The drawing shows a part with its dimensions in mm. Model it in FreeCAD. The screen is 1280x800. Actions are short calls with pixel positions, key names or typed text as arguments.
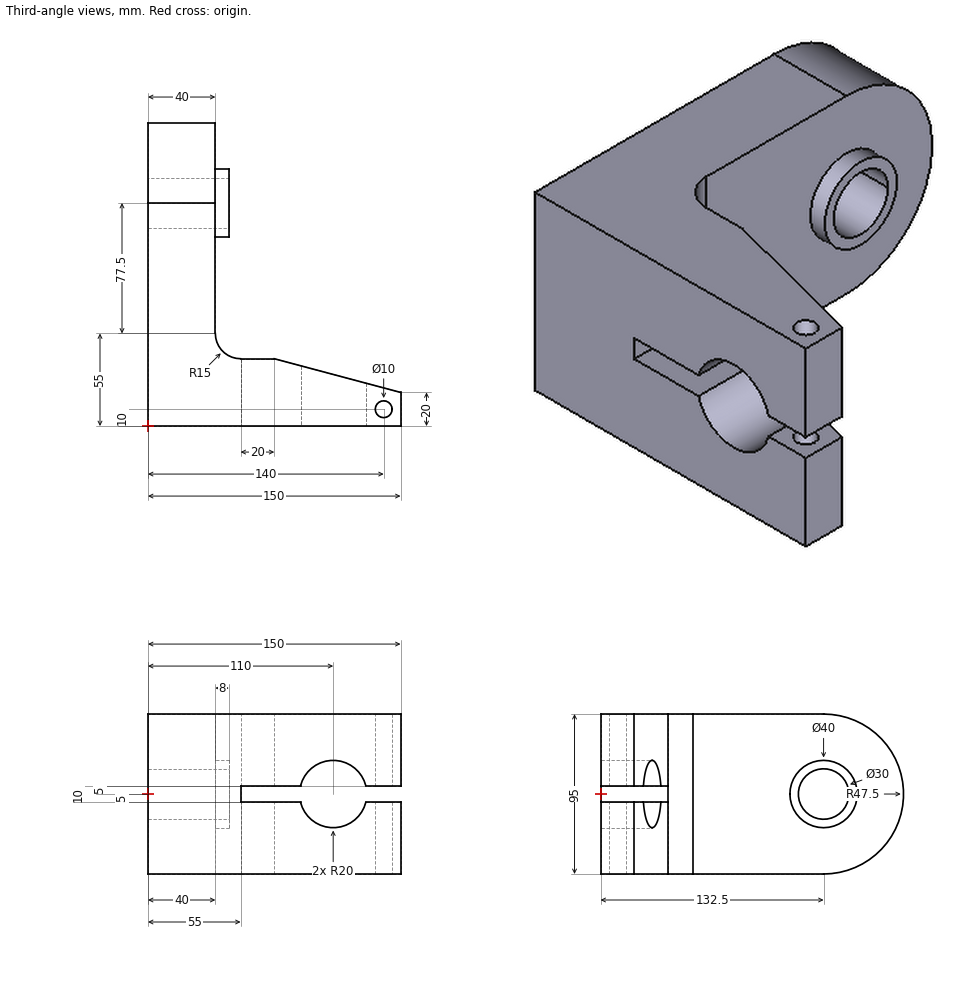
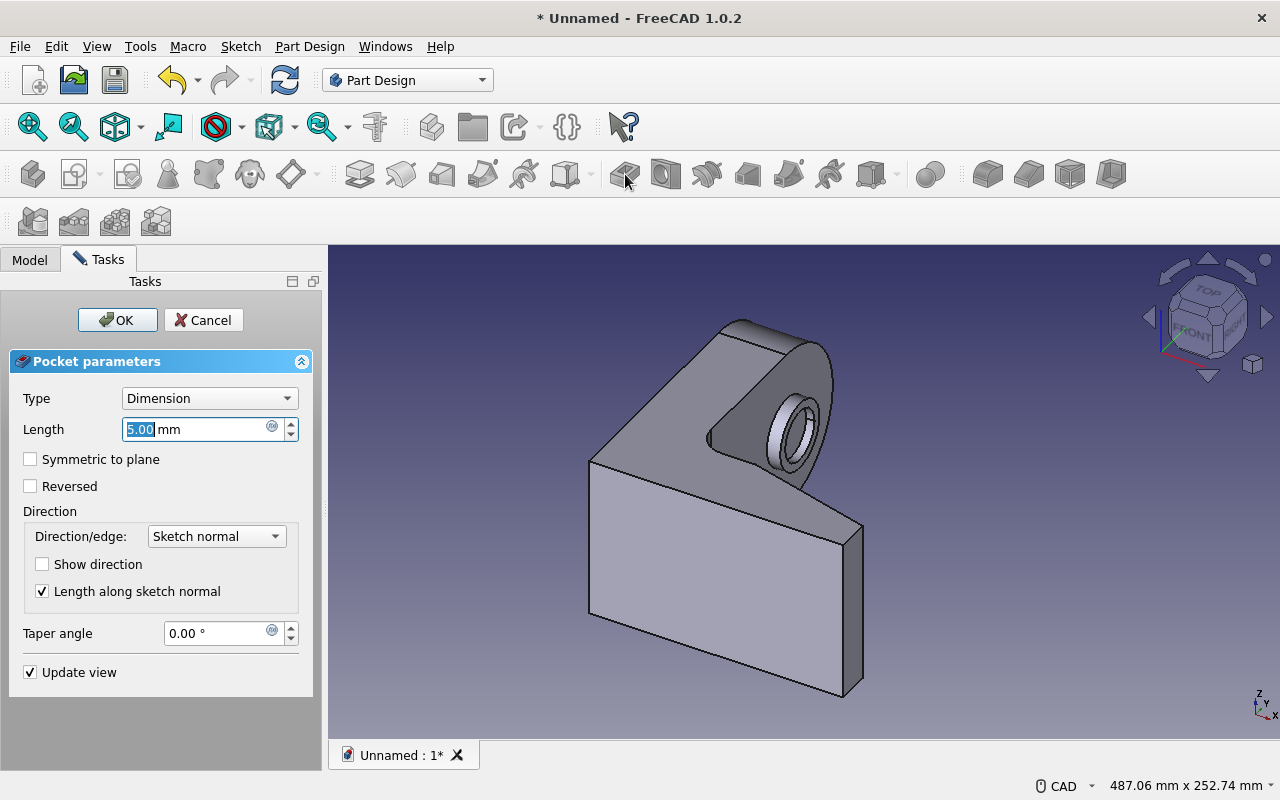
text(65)
key(Tab)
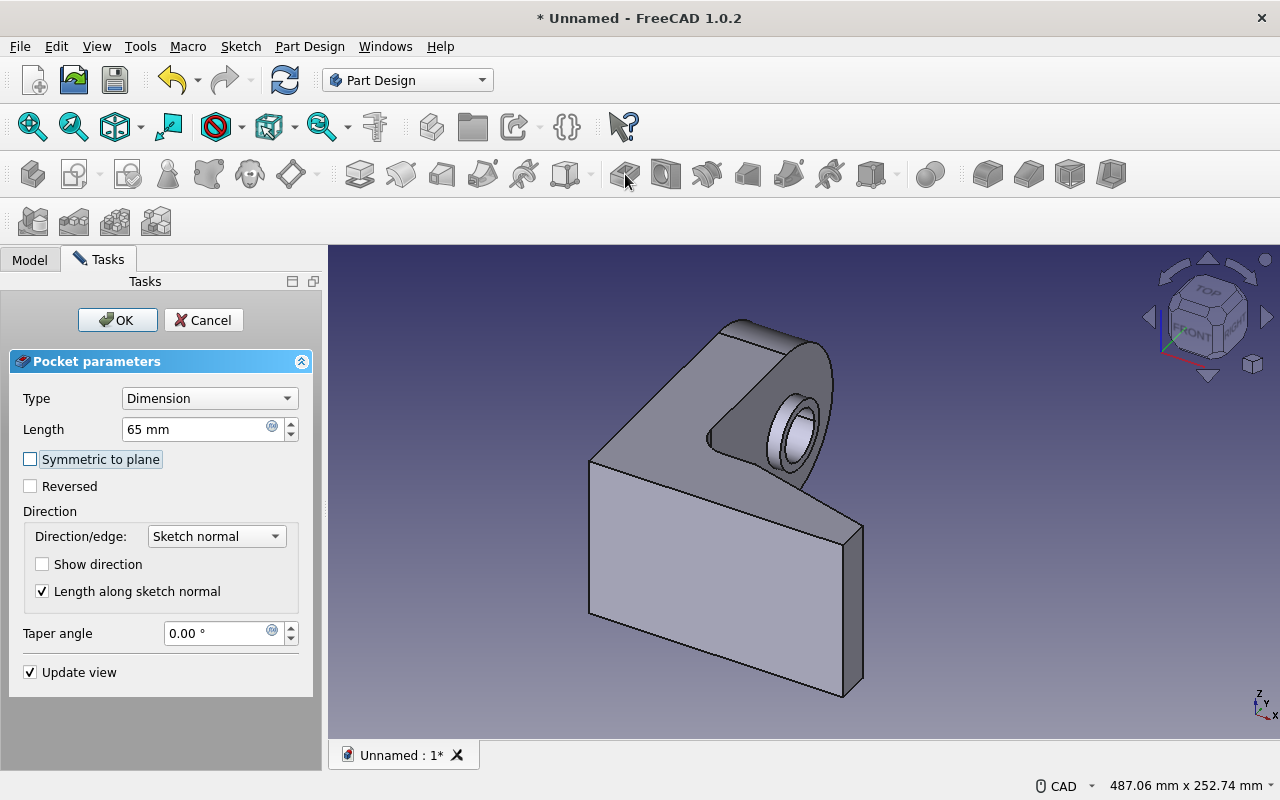
click(118, 320)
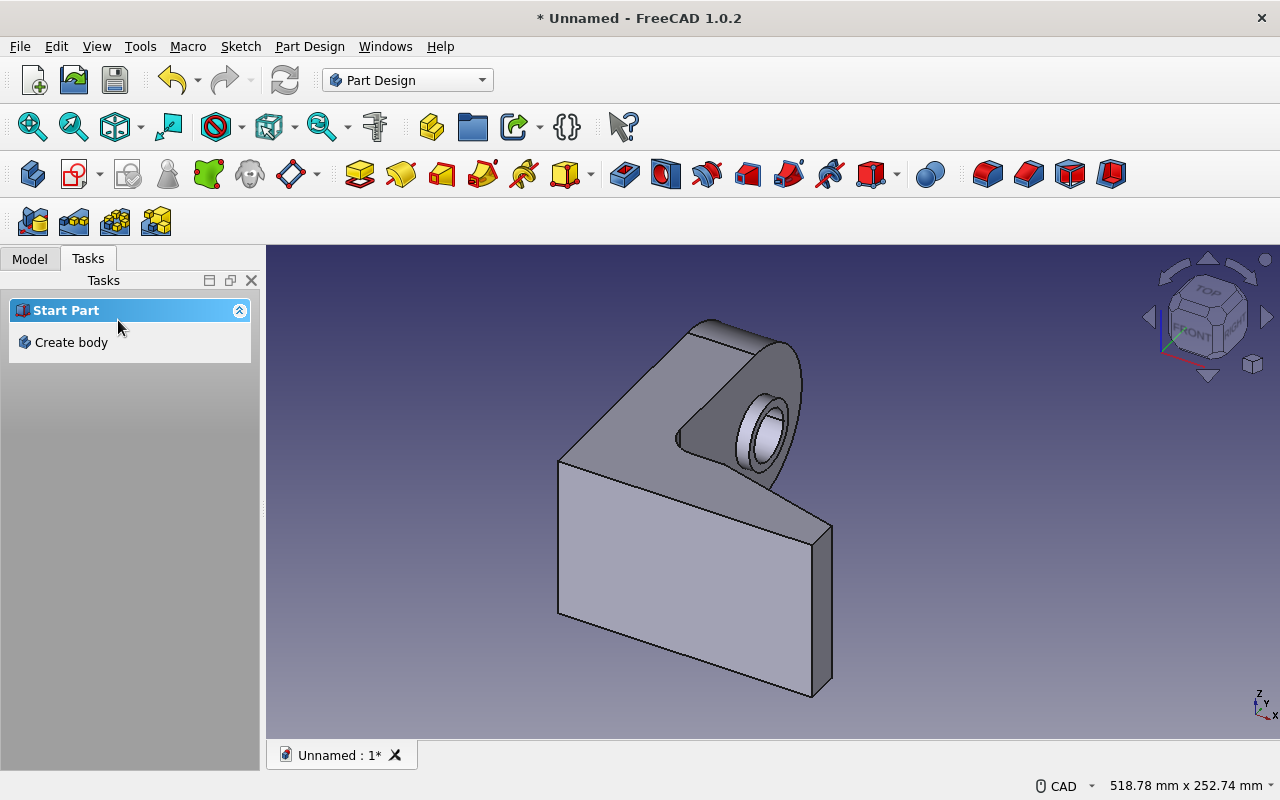
key(4)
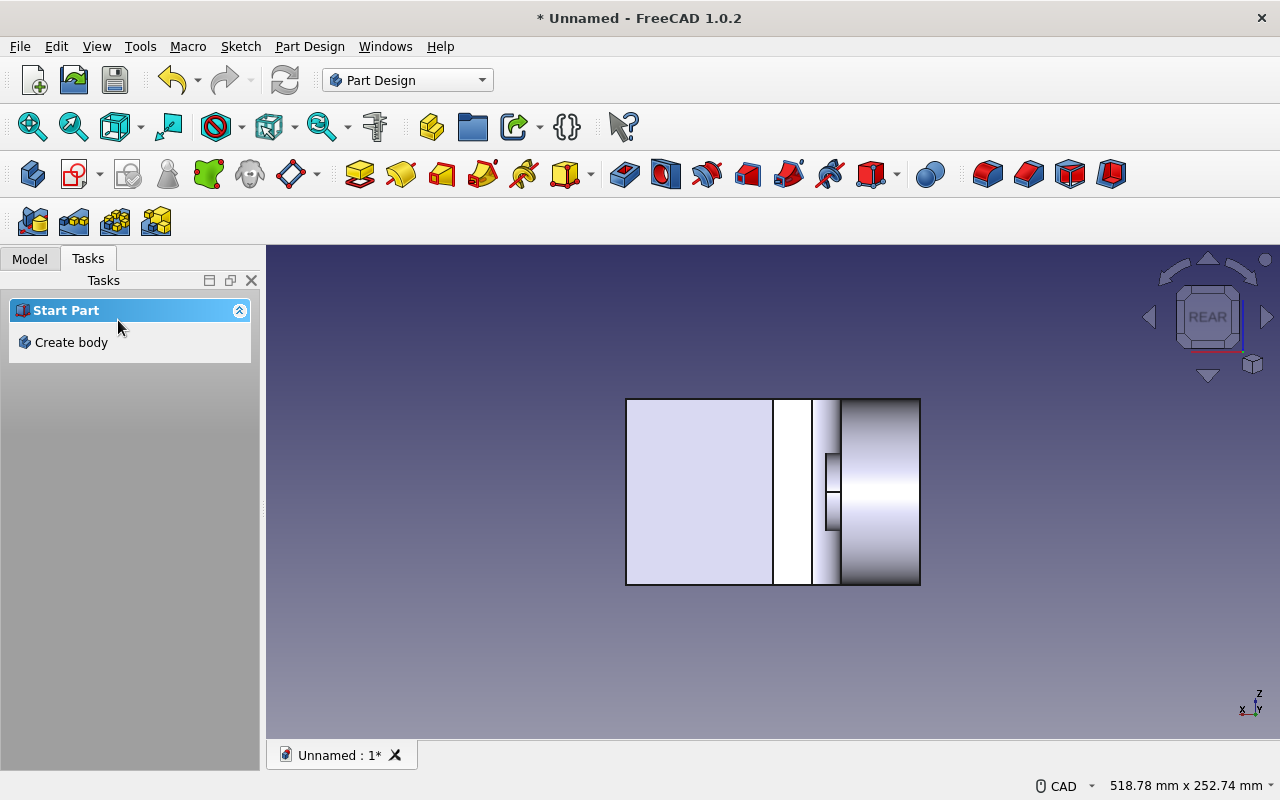
click(33, 128)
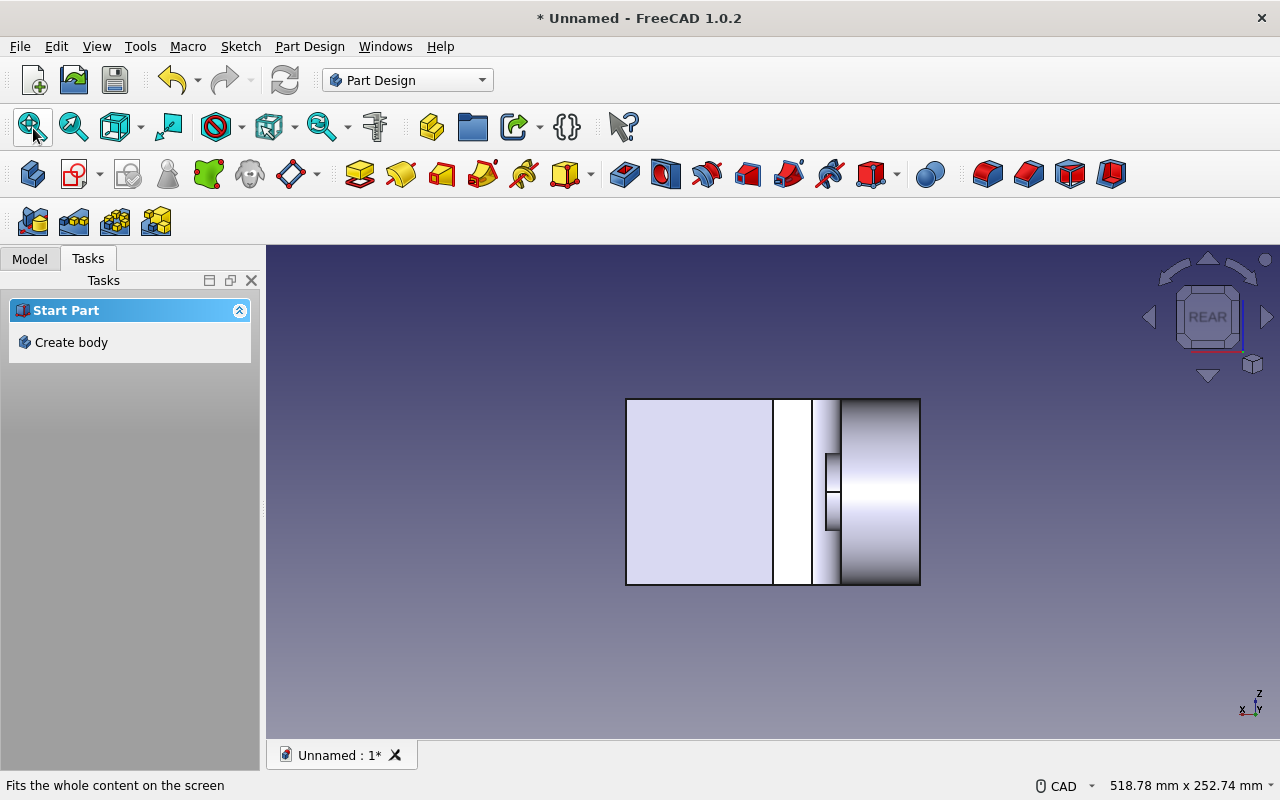
click(793, 438)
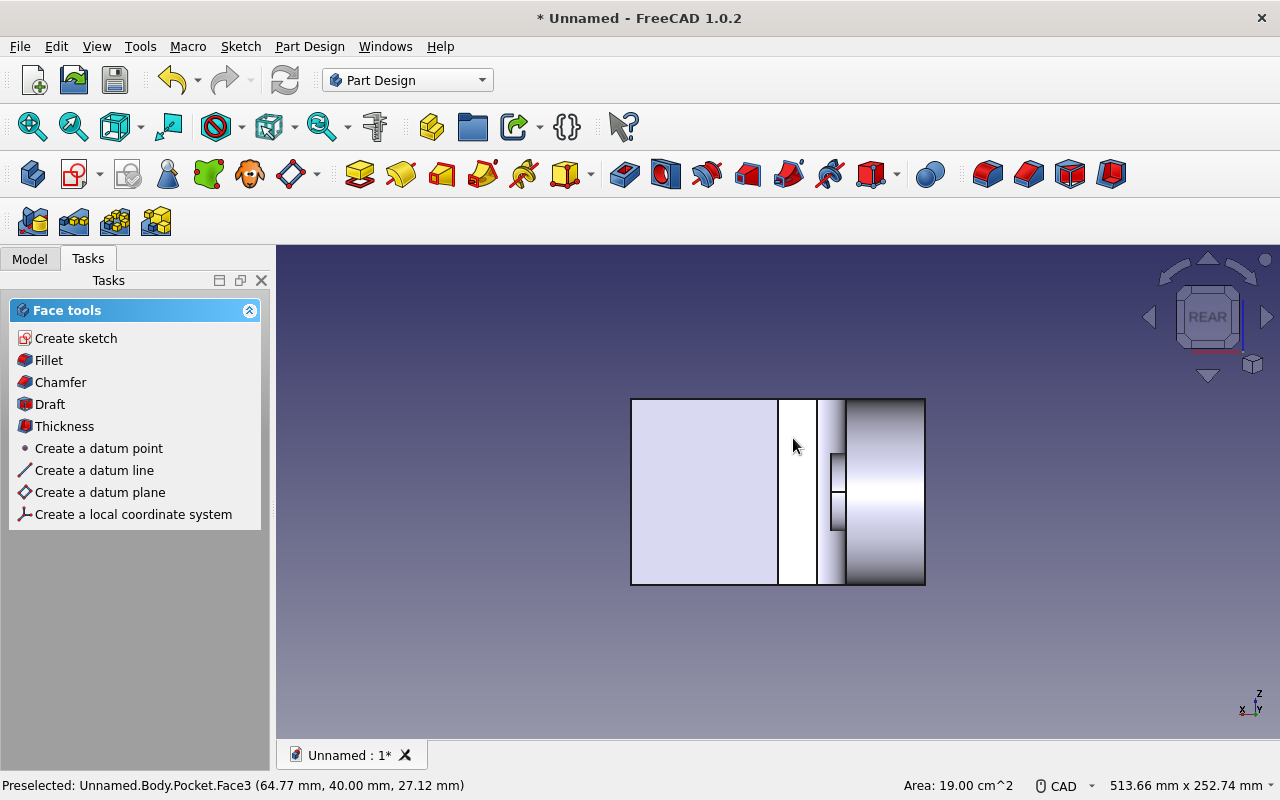
click(74, 174)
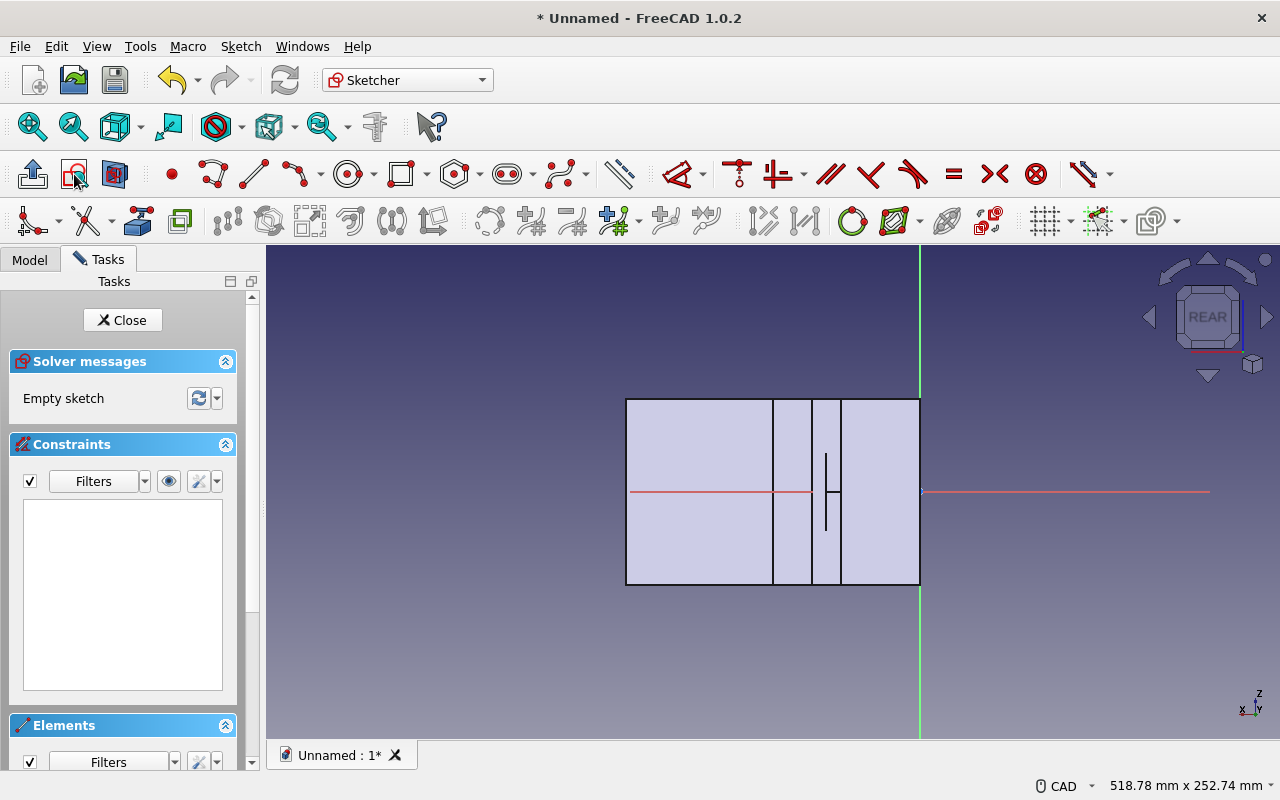
click(115, 174)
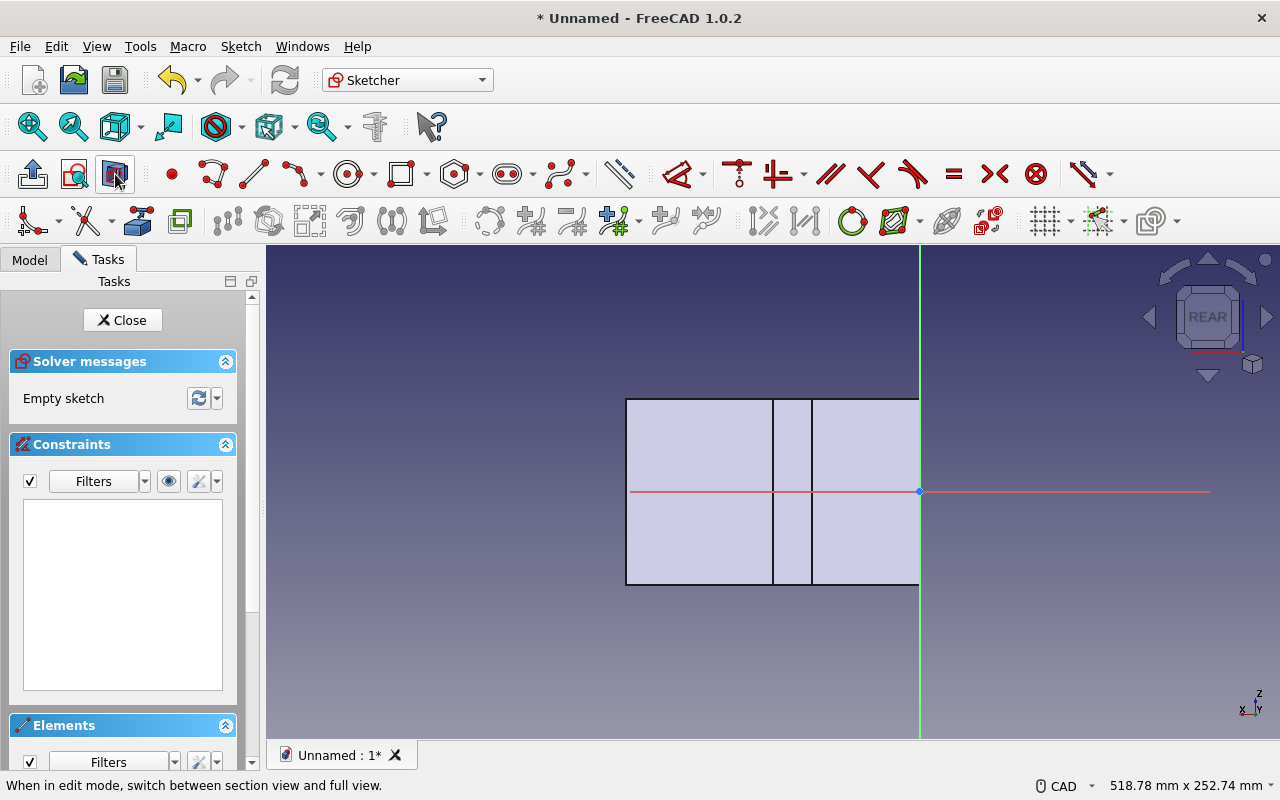
scroll(856, 492, up, 3)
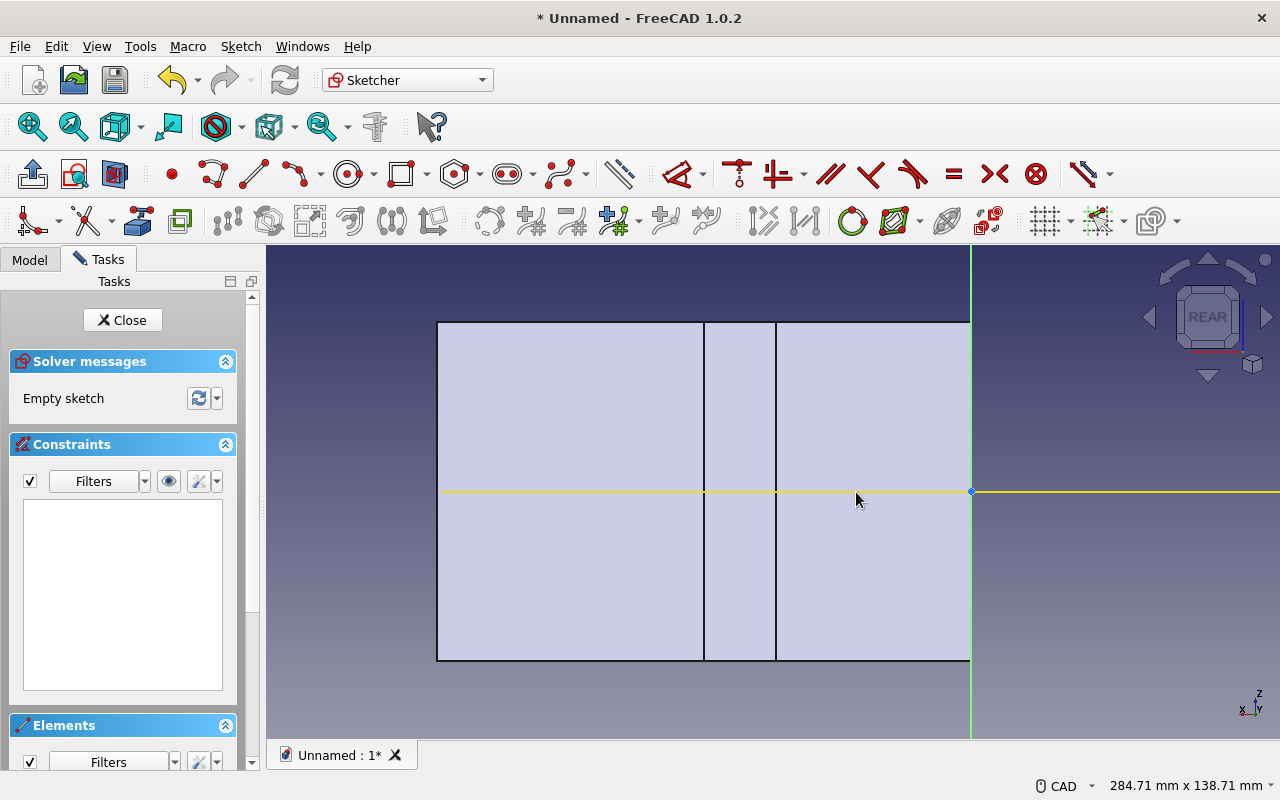
click(213, 174)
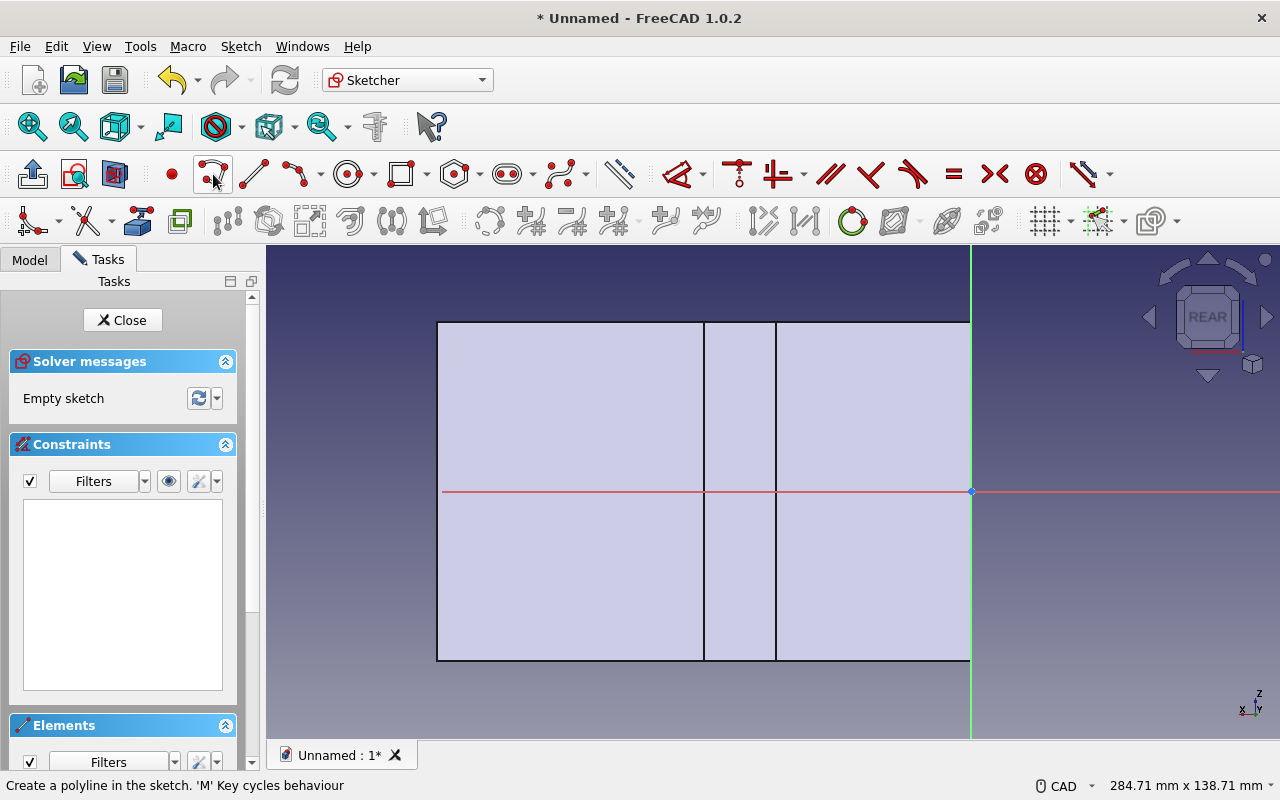
click(649, 509)
click(776, 509)
click(776, 474)
click(649, 474)
right_click(649, 474)